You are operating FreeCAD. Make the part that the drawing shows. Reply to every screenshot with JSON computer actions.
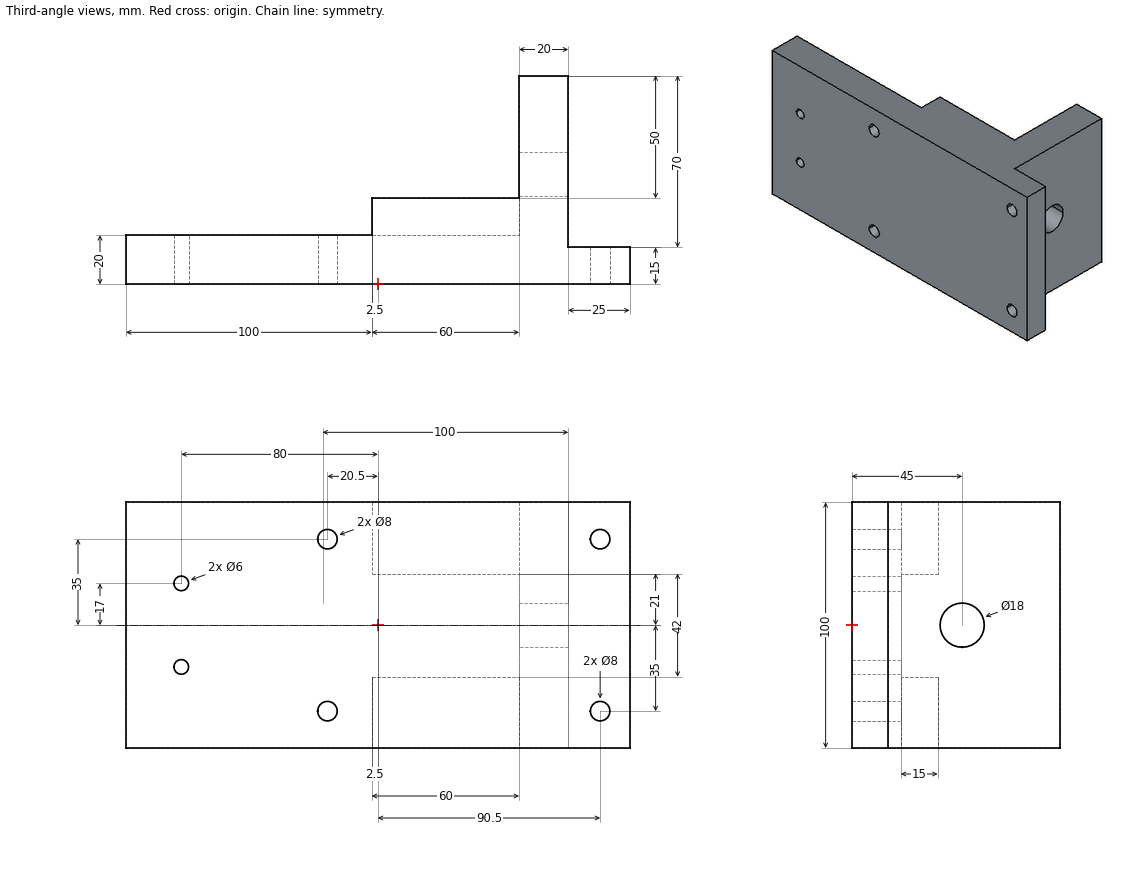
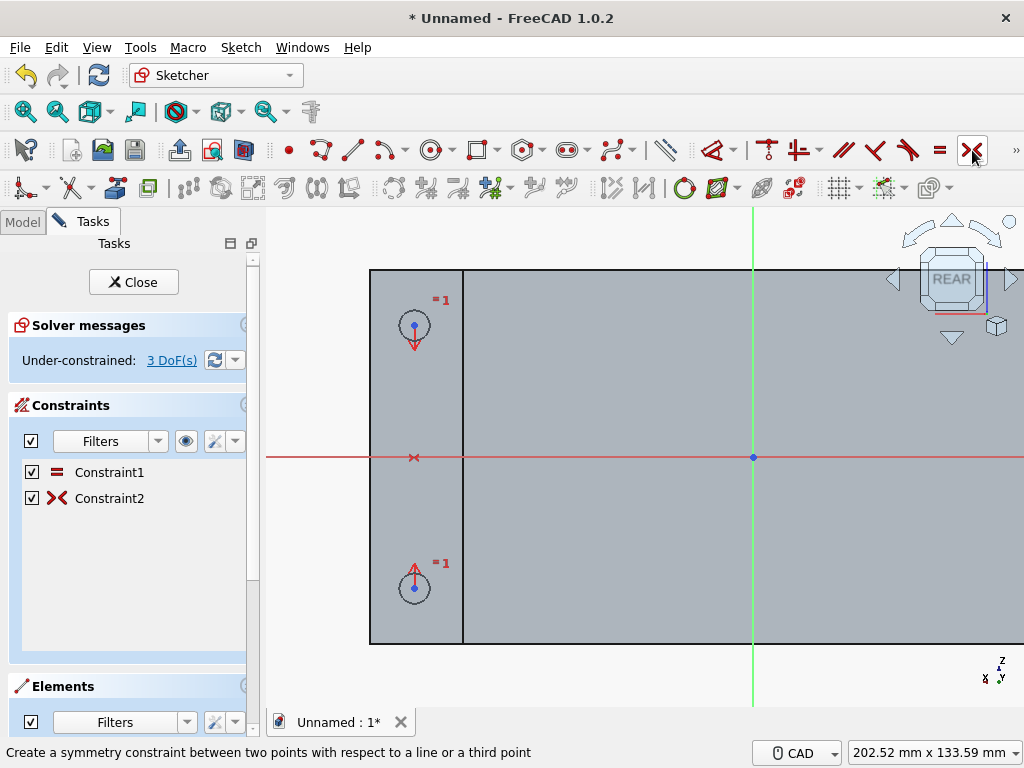
{"action": "left_click", "coordinate": [712, 150]}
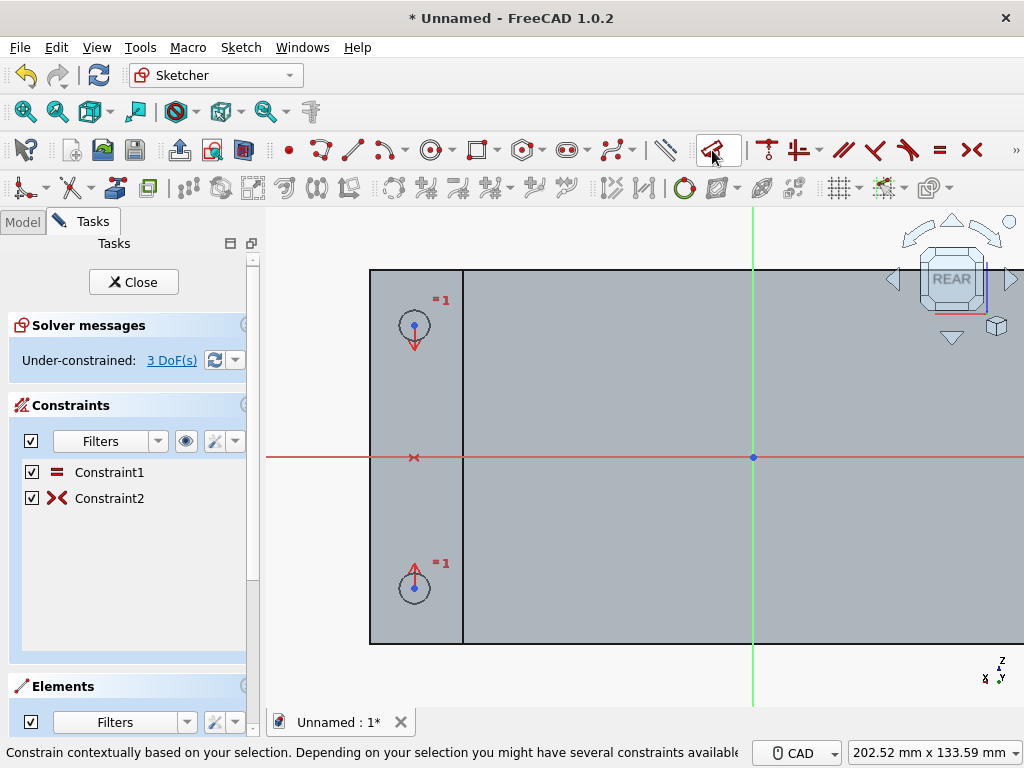
{"action": "scroll", "coordinate": [425, 578], "scroll_direction": "up", "scroll_amount": 2}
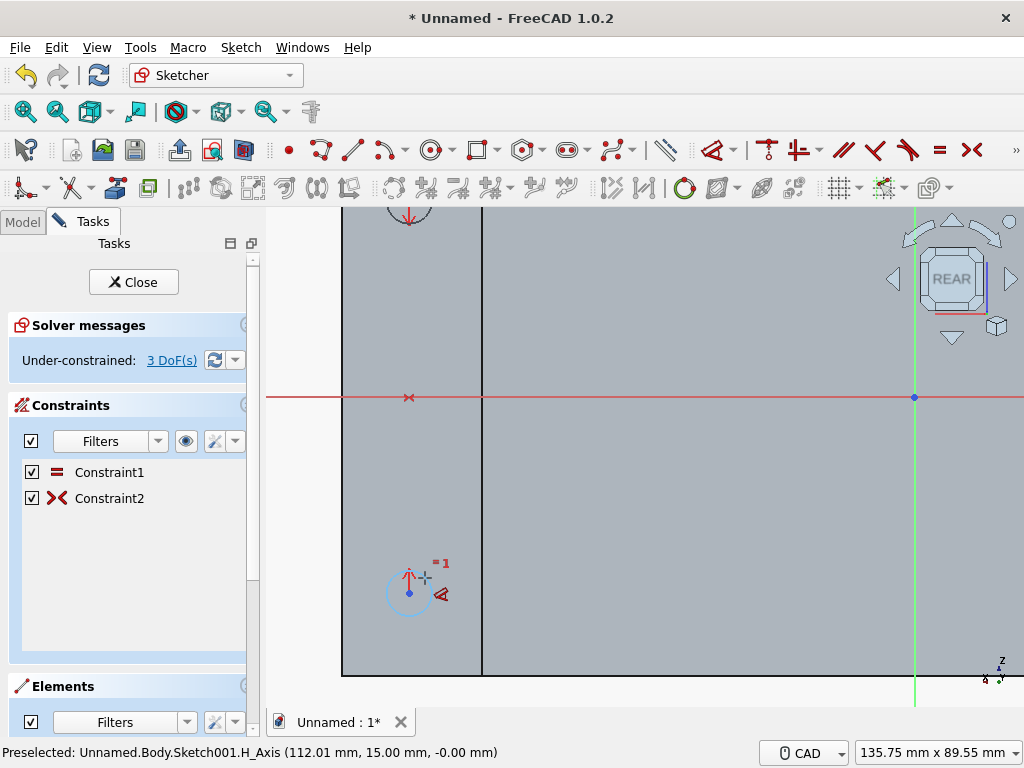
{"action": "left_click", "coordinate": [425, 577]}
{"action": "left_click", "coordinate": [447, 554]}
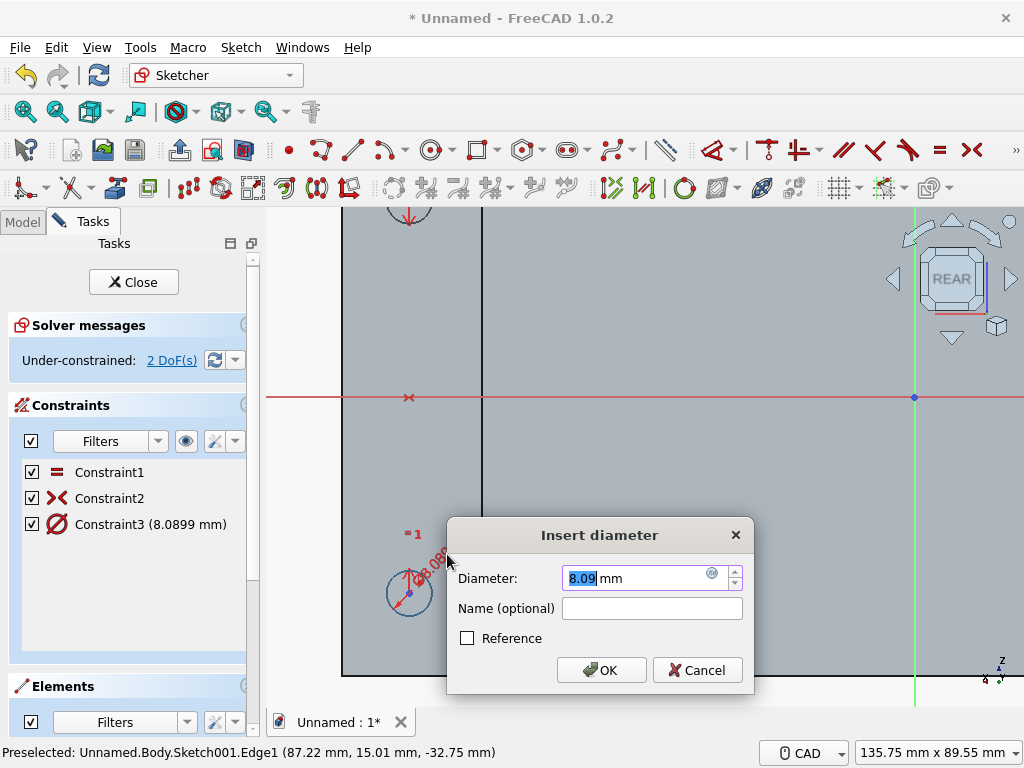
{"action": "type", "text": "8"}
{"action": "key", "text": "Return"}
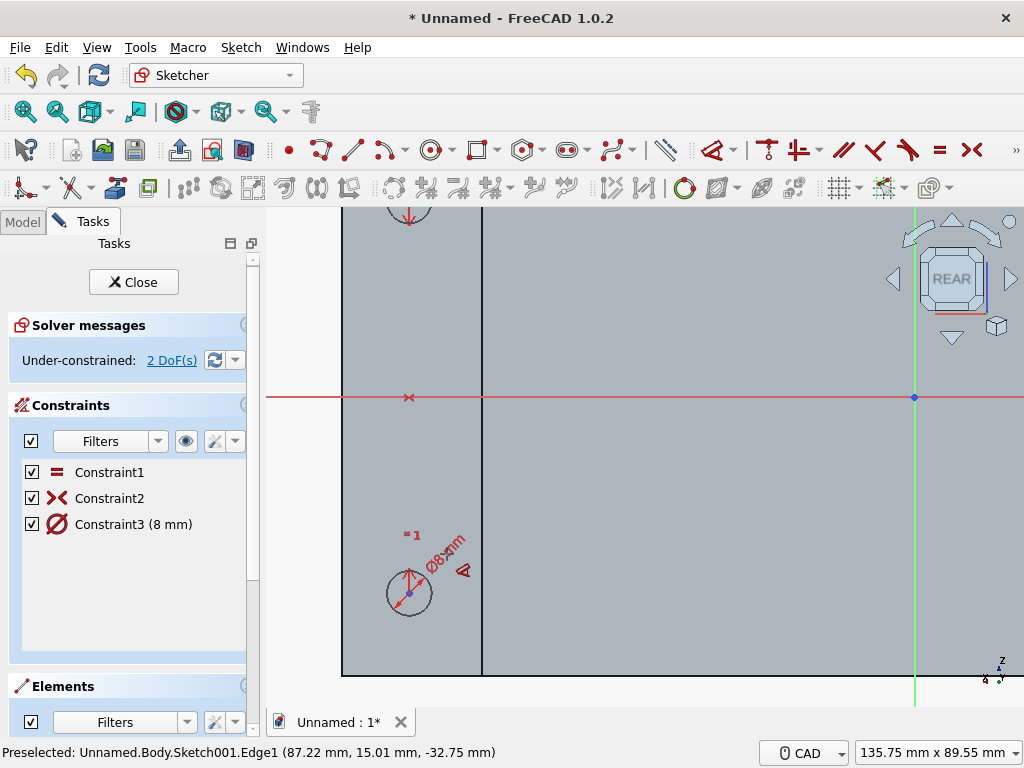
{"action": "left_click", "coordinate": [409, 593]}
{"action": "left_click", "coordinate": [375, 495]}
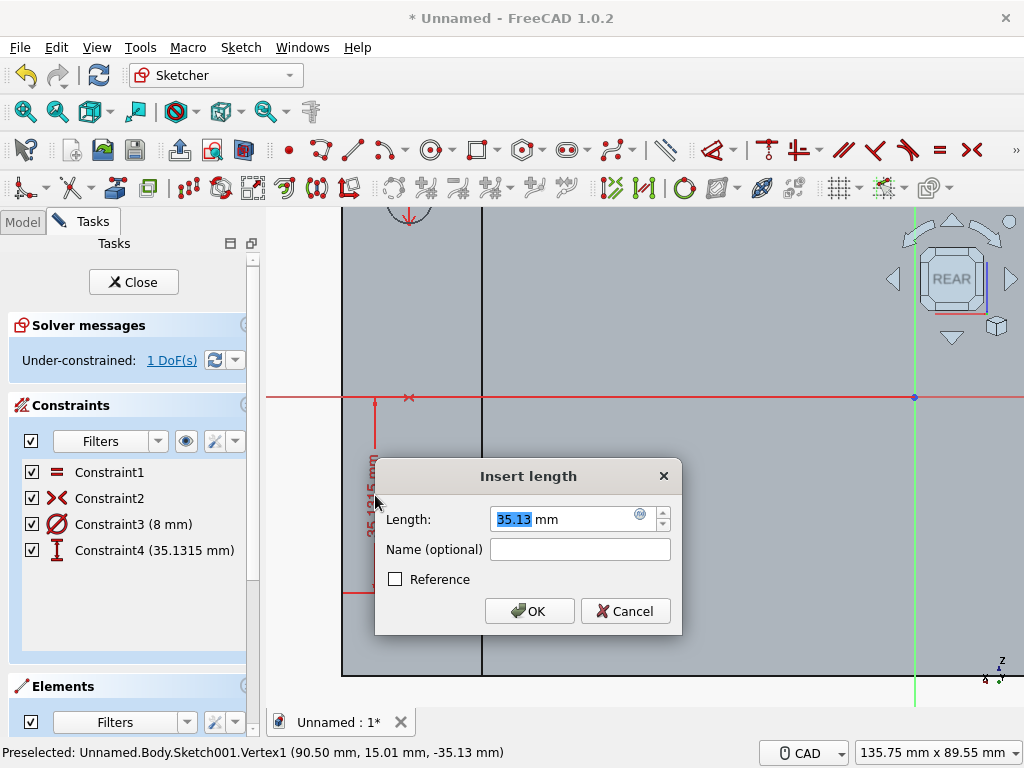
{"action": "type", "text": "35"}
{"action": "key", "text": "Return"}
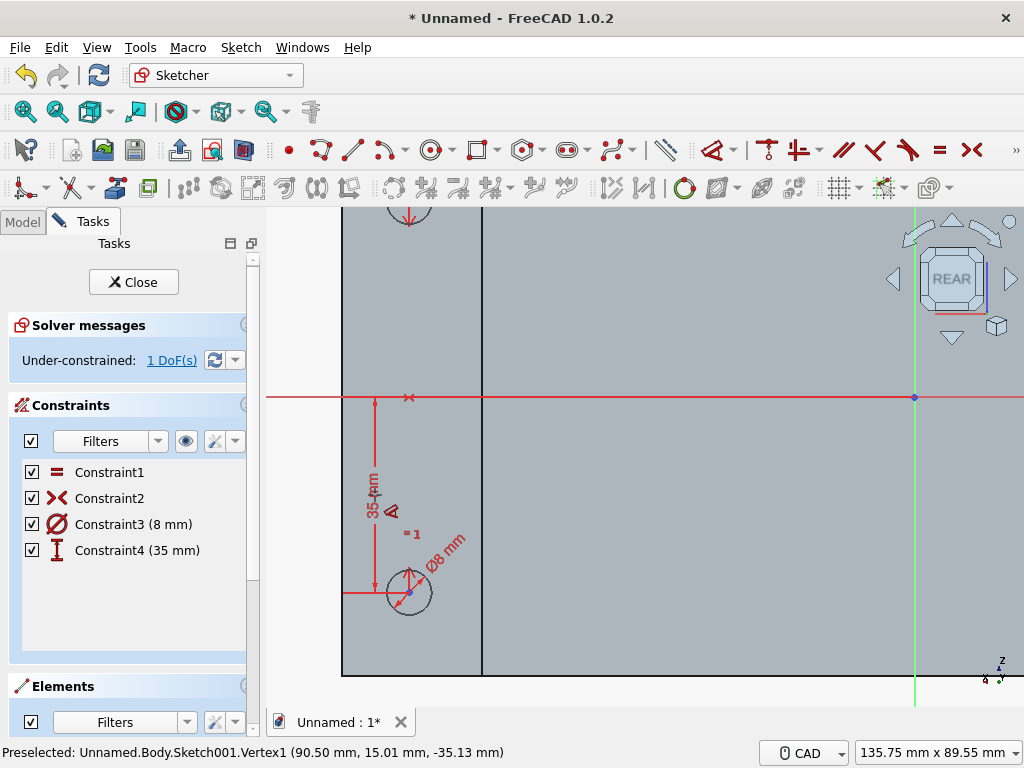
{"action": "left_click", "coordinate": [409, 593]}
{"action": "left_click", "coordinate": [634, 627]}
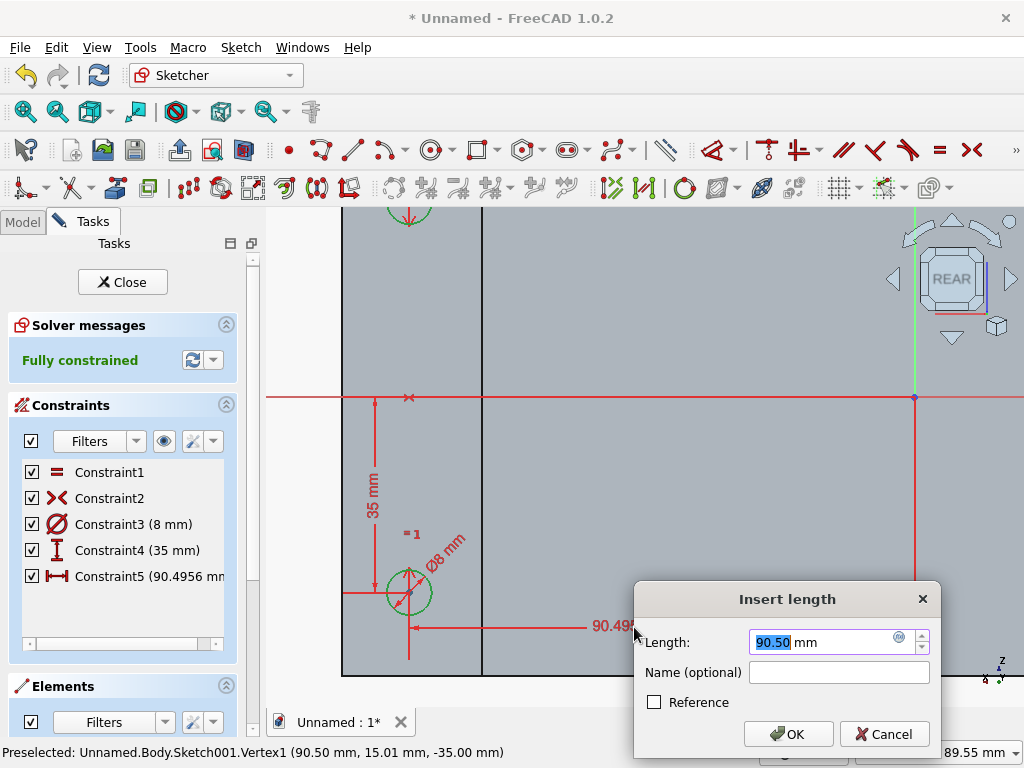
{"action": "type", "text": "90.5"}
{"action": "key", "text": "Return"}
{"action": "key", "text": "Escape"}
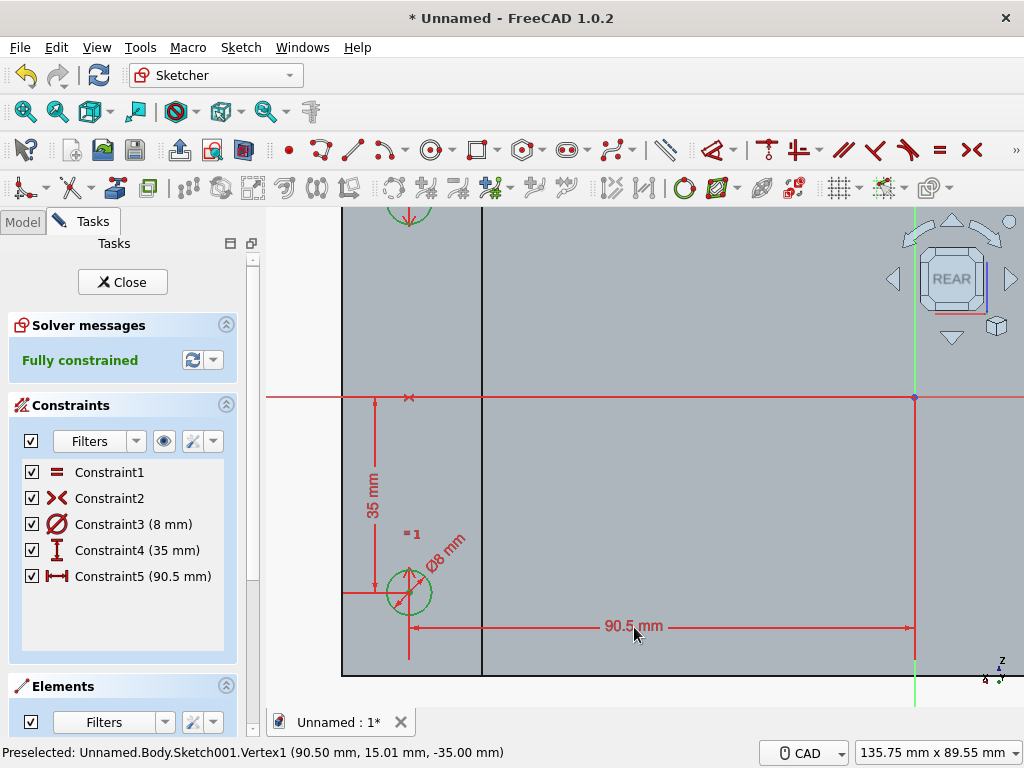
{"action": "left_click", "coordinate": [123, 282]}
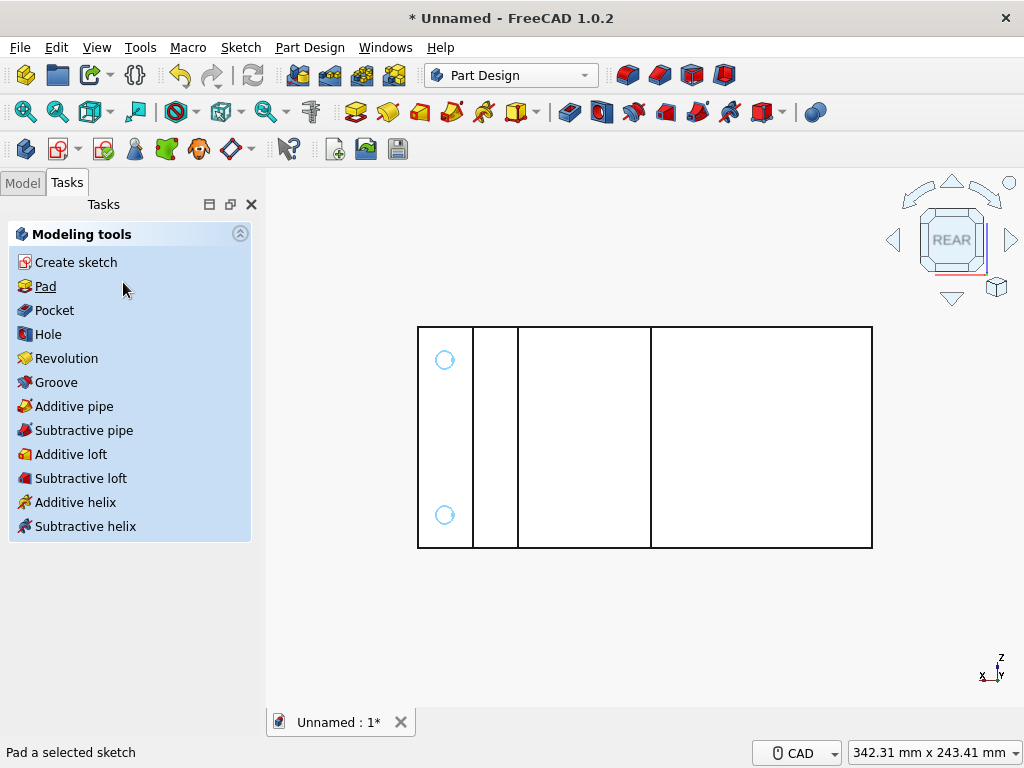
{"action": "left_click", "coordinate": [570, 112]}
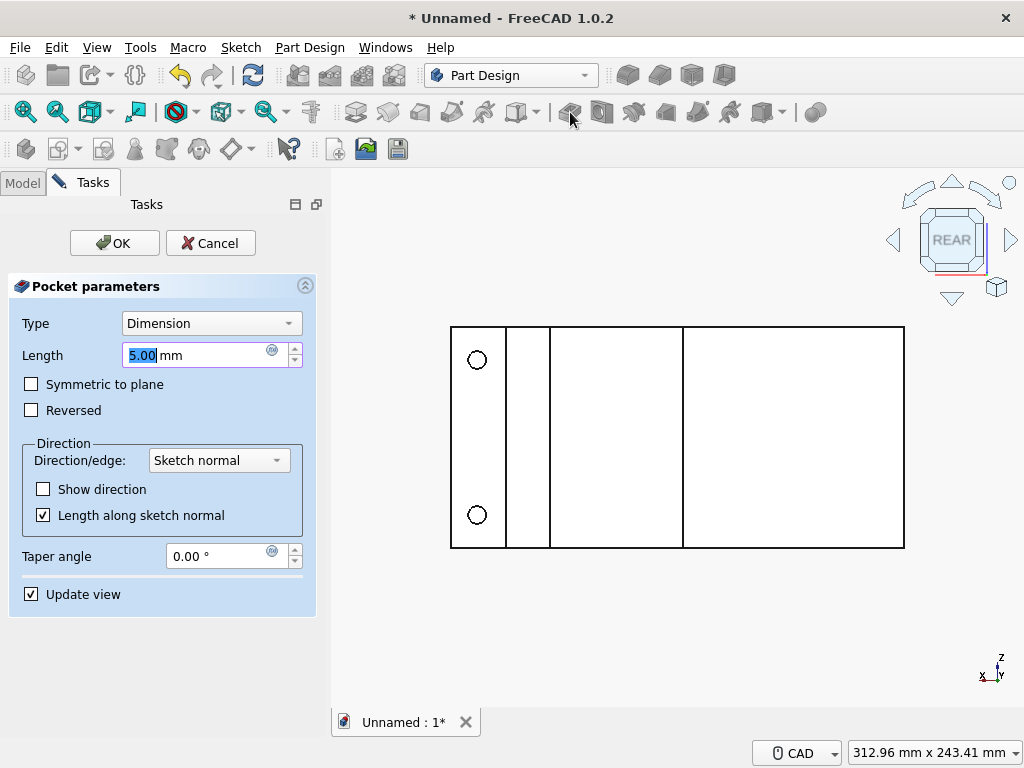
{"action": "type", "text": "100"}
{"action": "key", "text": "Tab"}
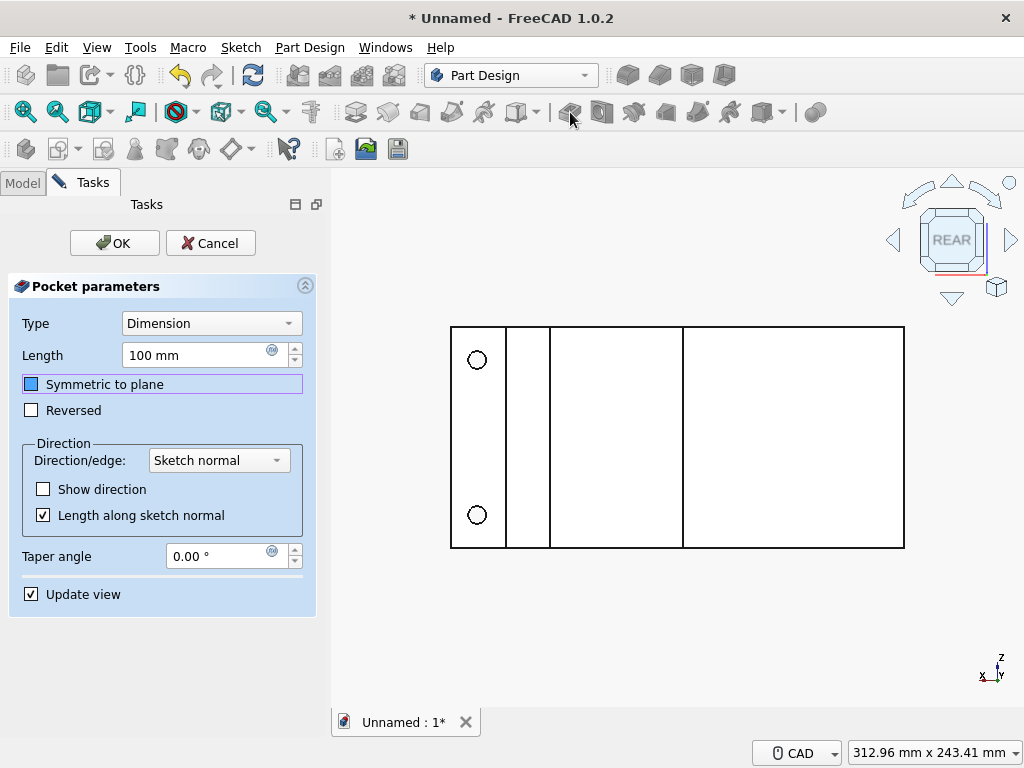
{"action": "left_click", "coordinate": [115, 243]}